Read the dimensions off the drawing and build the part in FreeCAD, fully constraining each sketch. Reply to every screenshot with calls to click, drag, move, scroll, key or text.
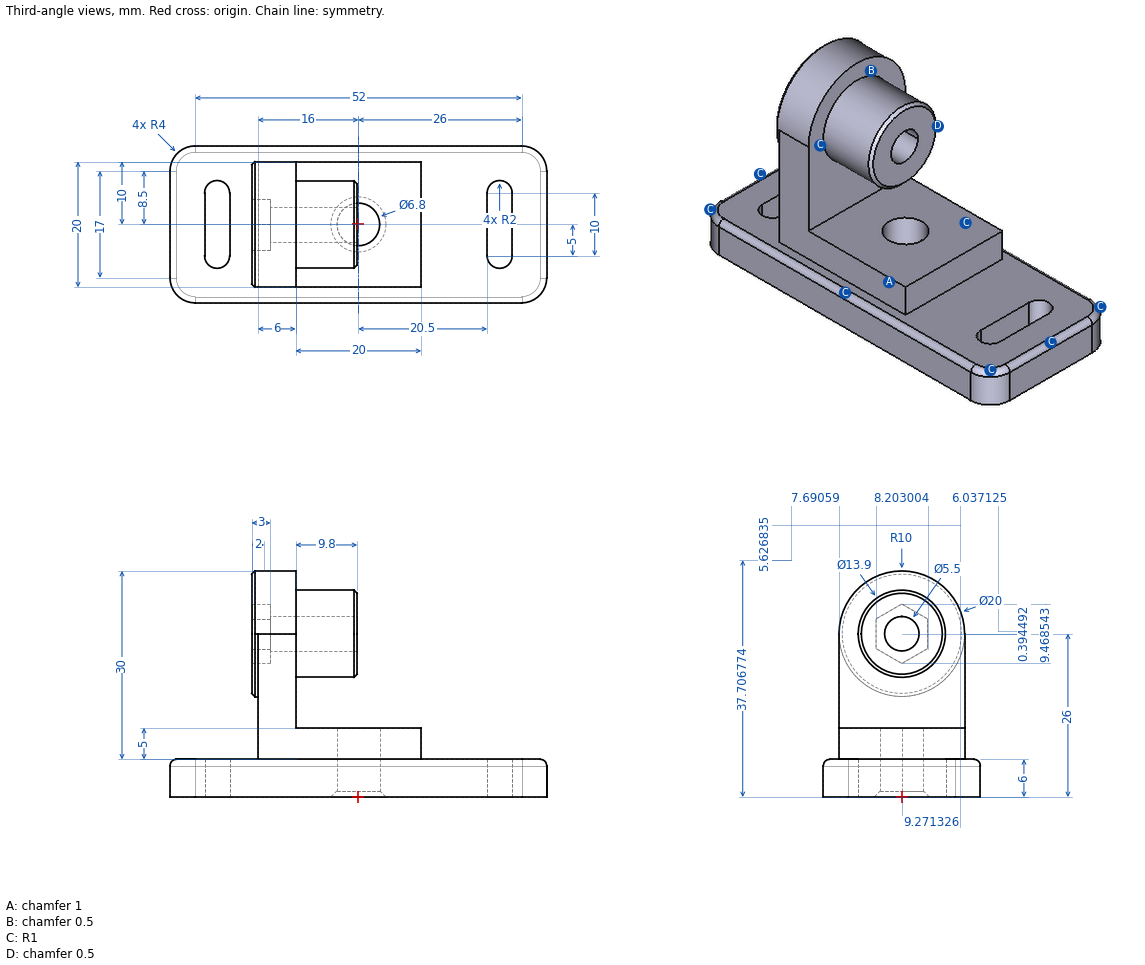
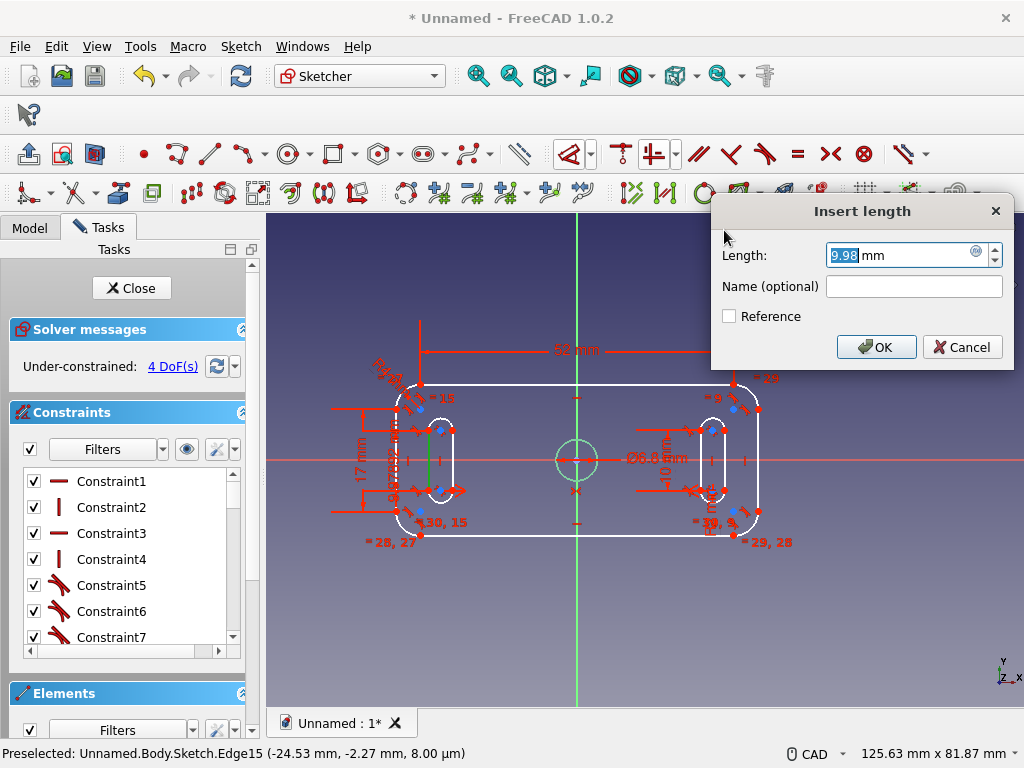
text(10)
key(Return)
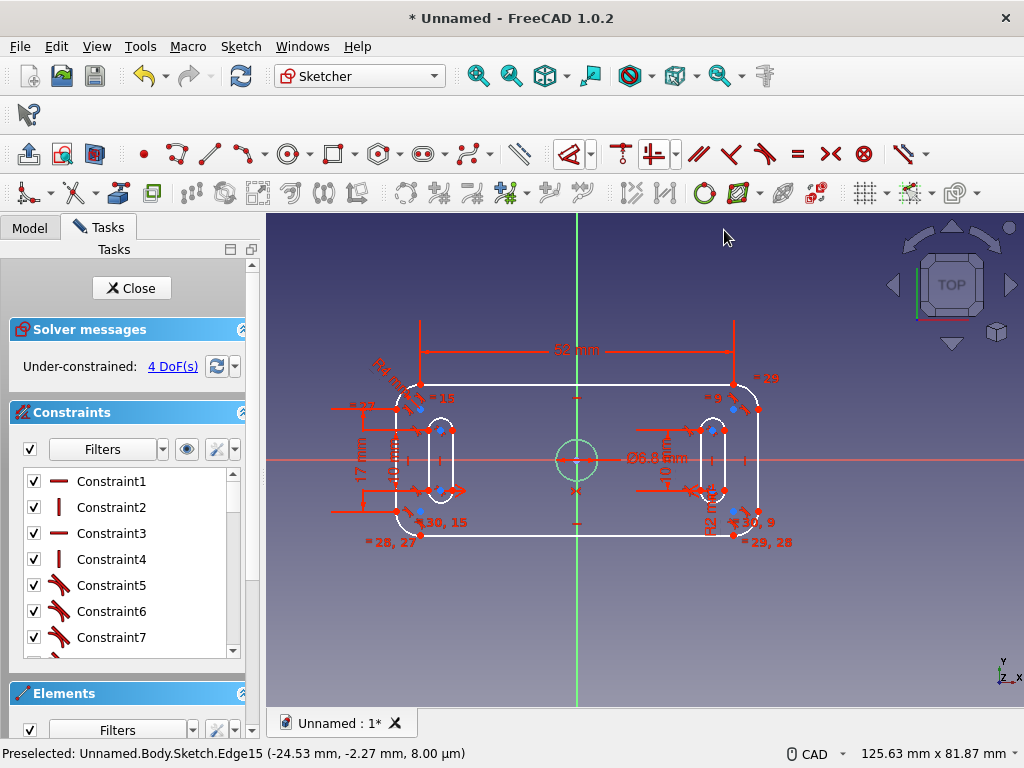
scroll(701, 491, up, 2)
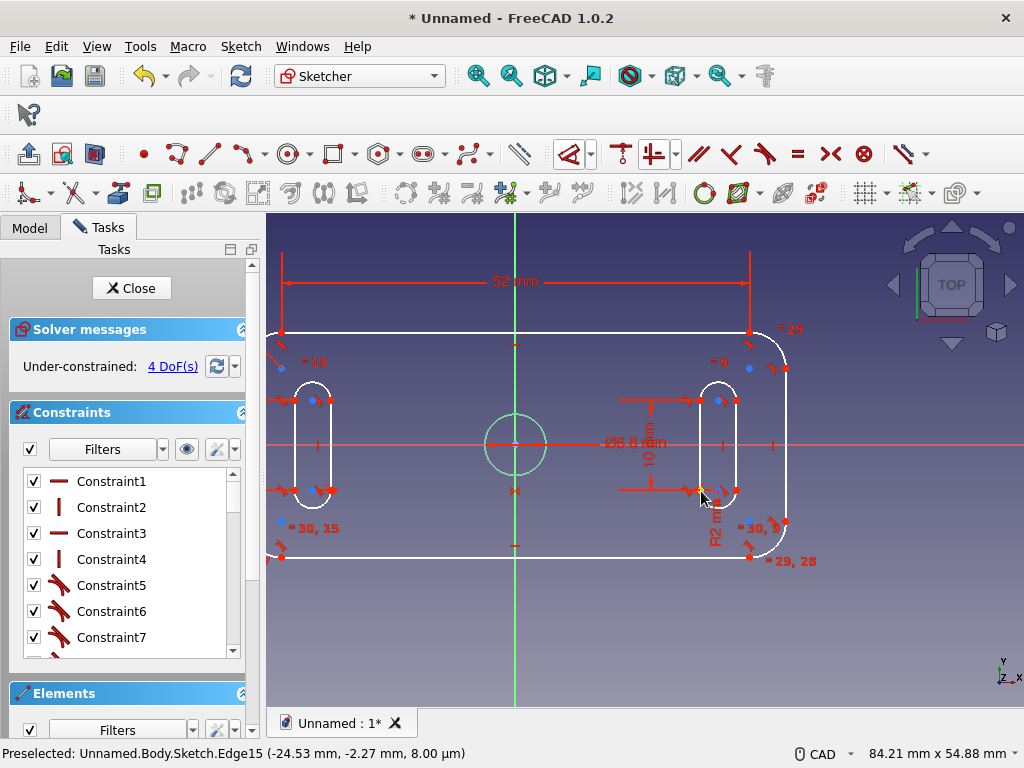
click(700, 490)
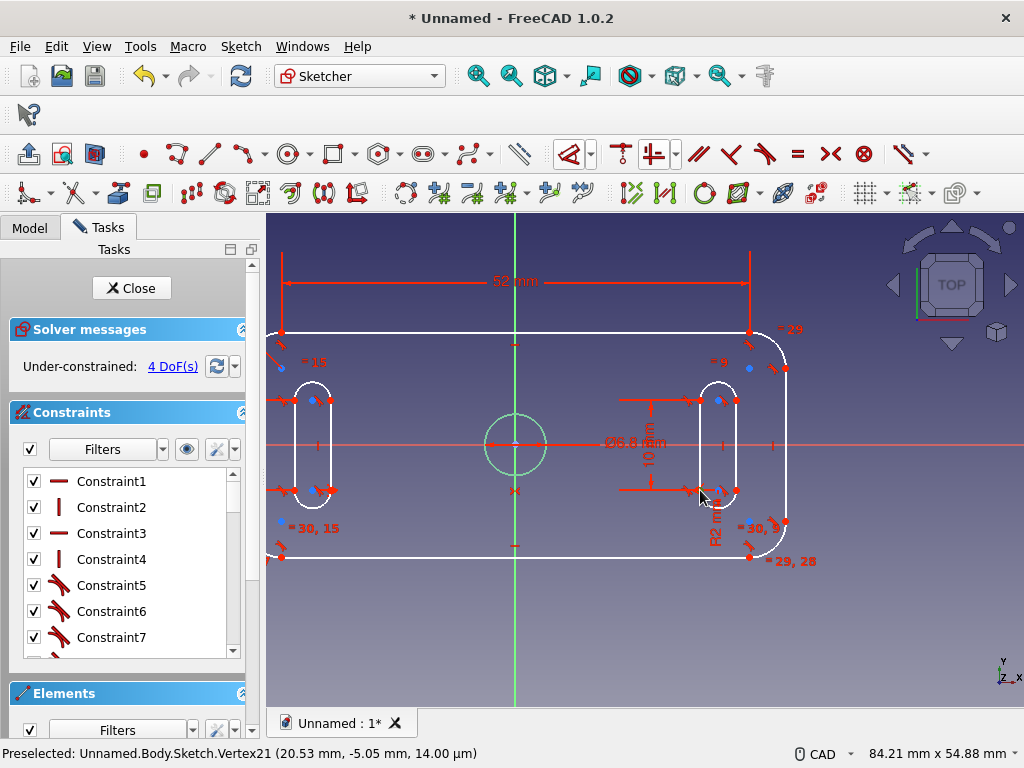
key(i)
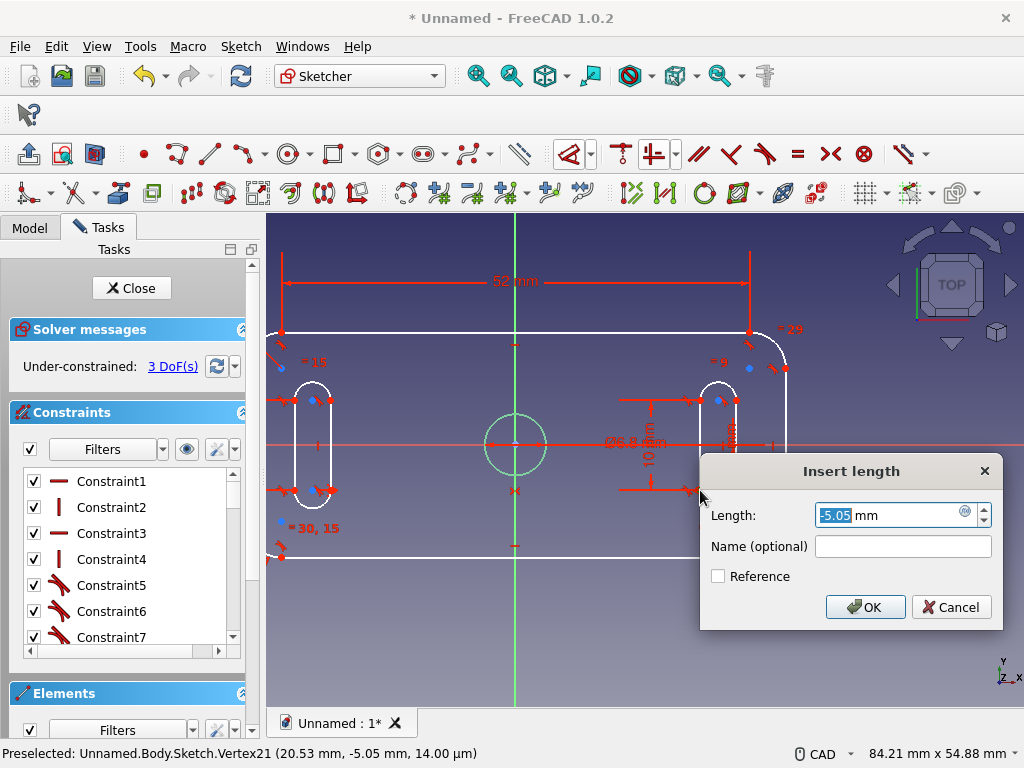
text(-5)
key(Return)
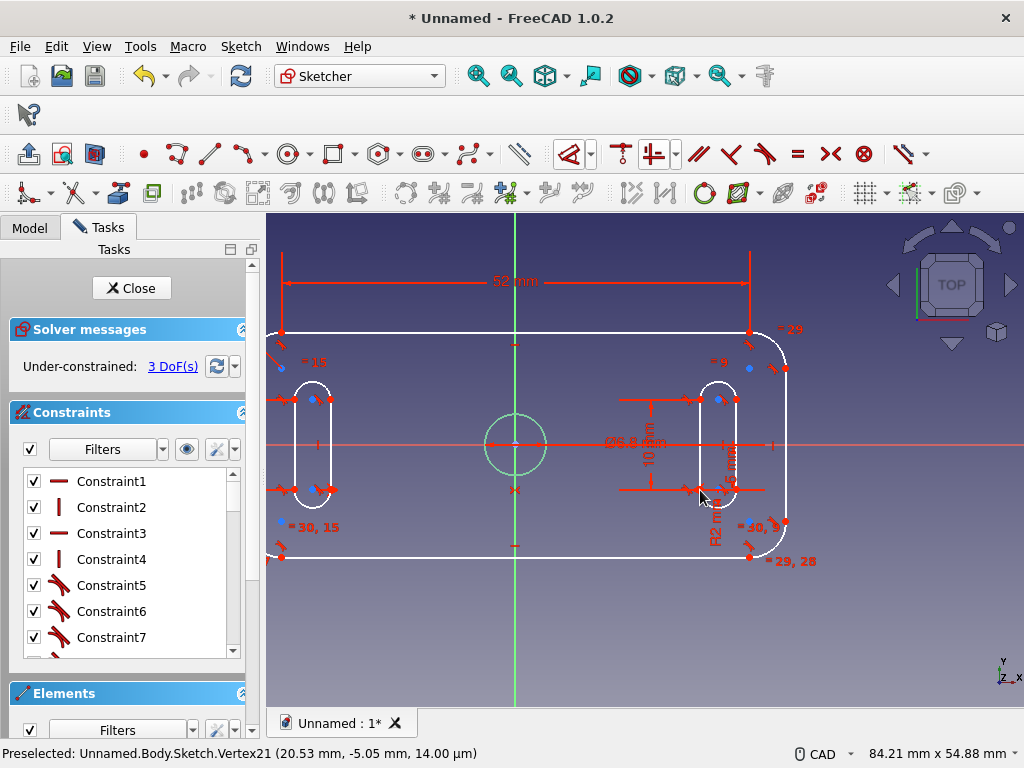
click(750, 333)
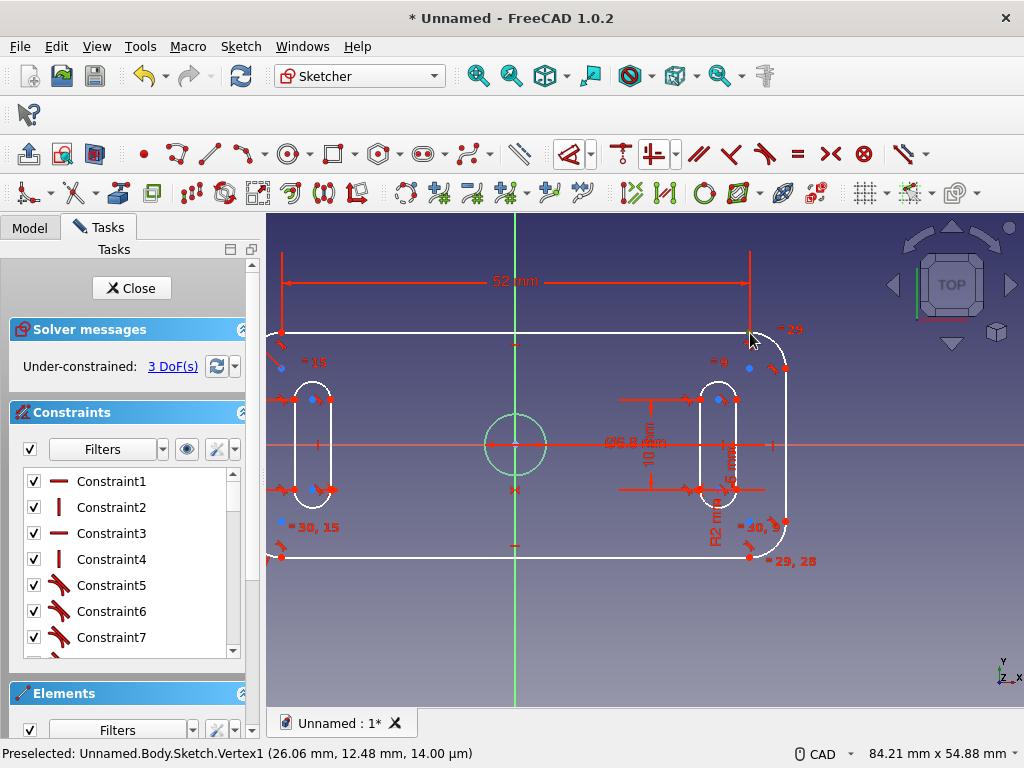
key(l)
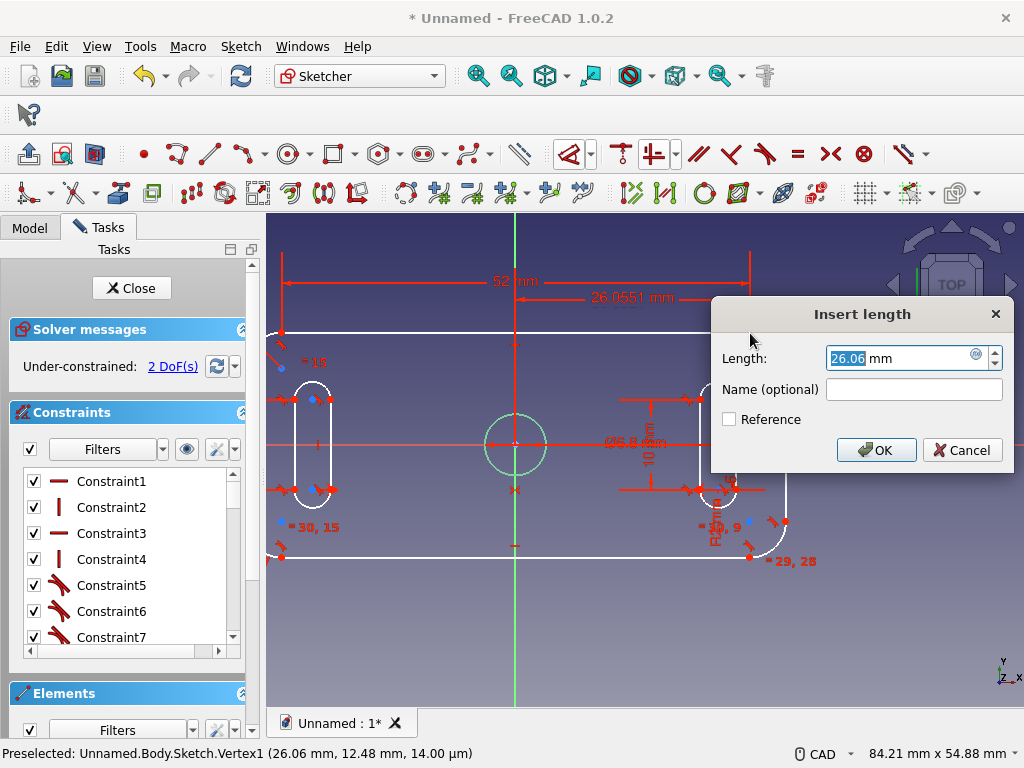
text(26)
key(Return)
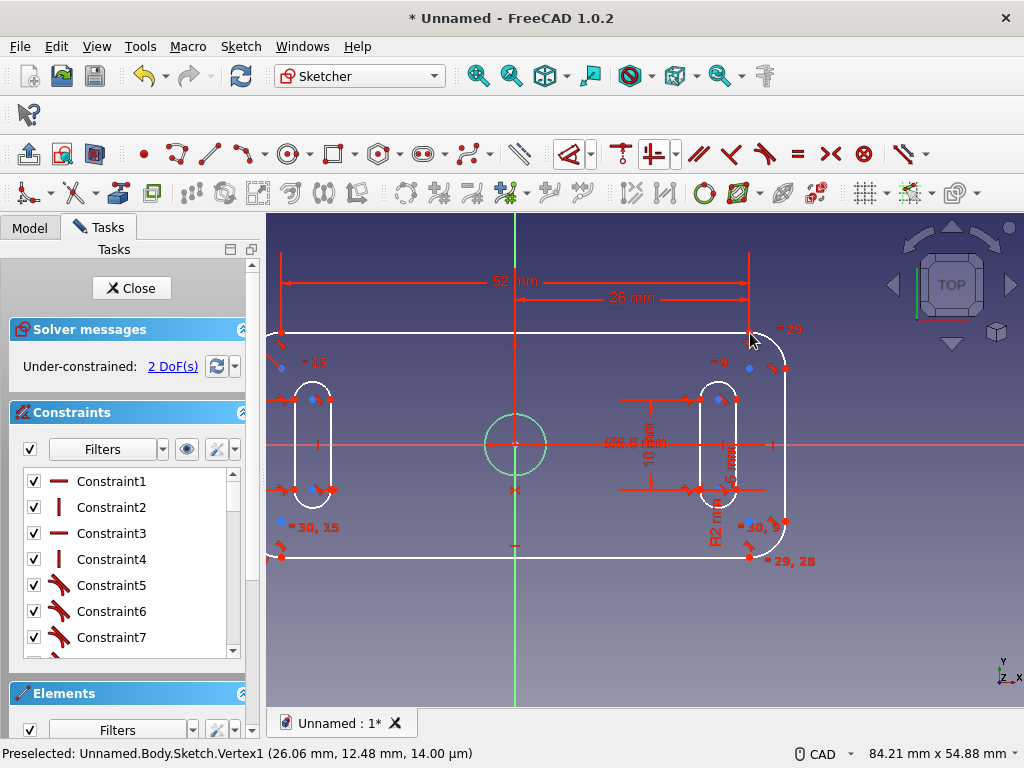
scroll(701, 491, down, 2)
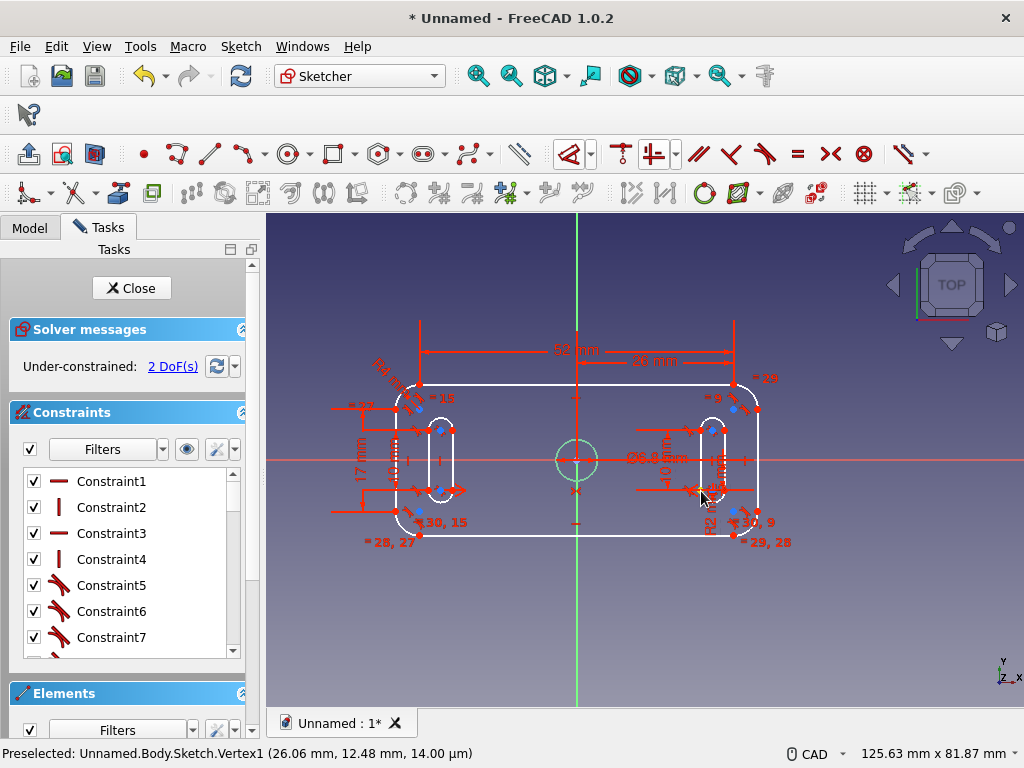
click(396, 409)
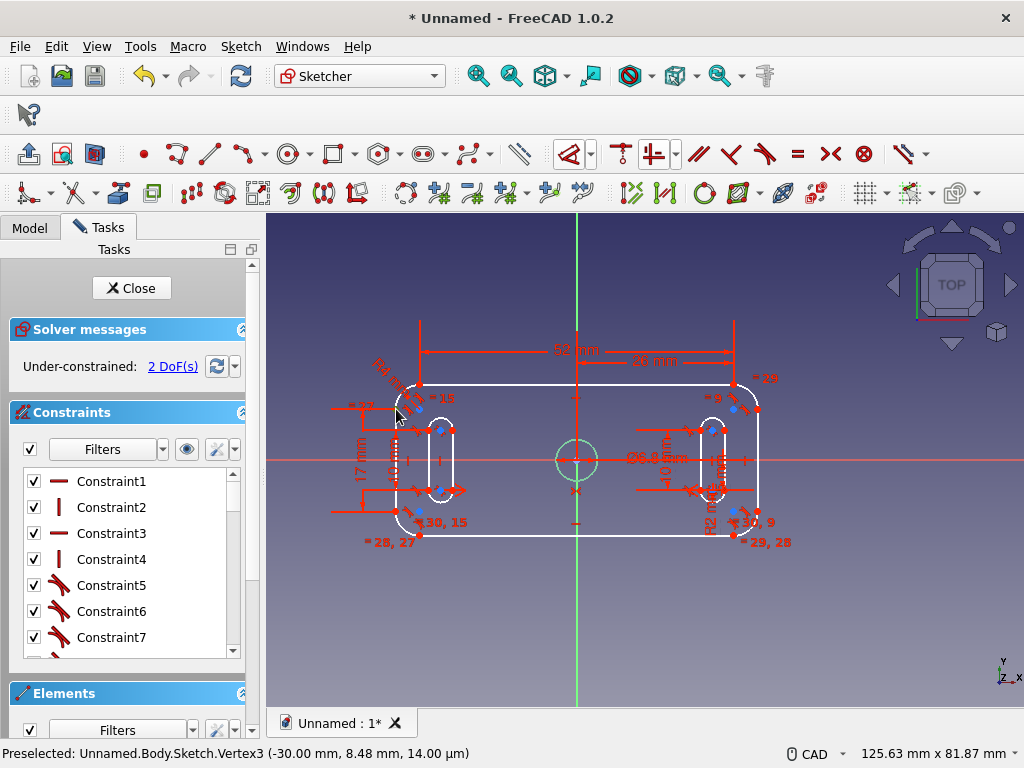
key(i)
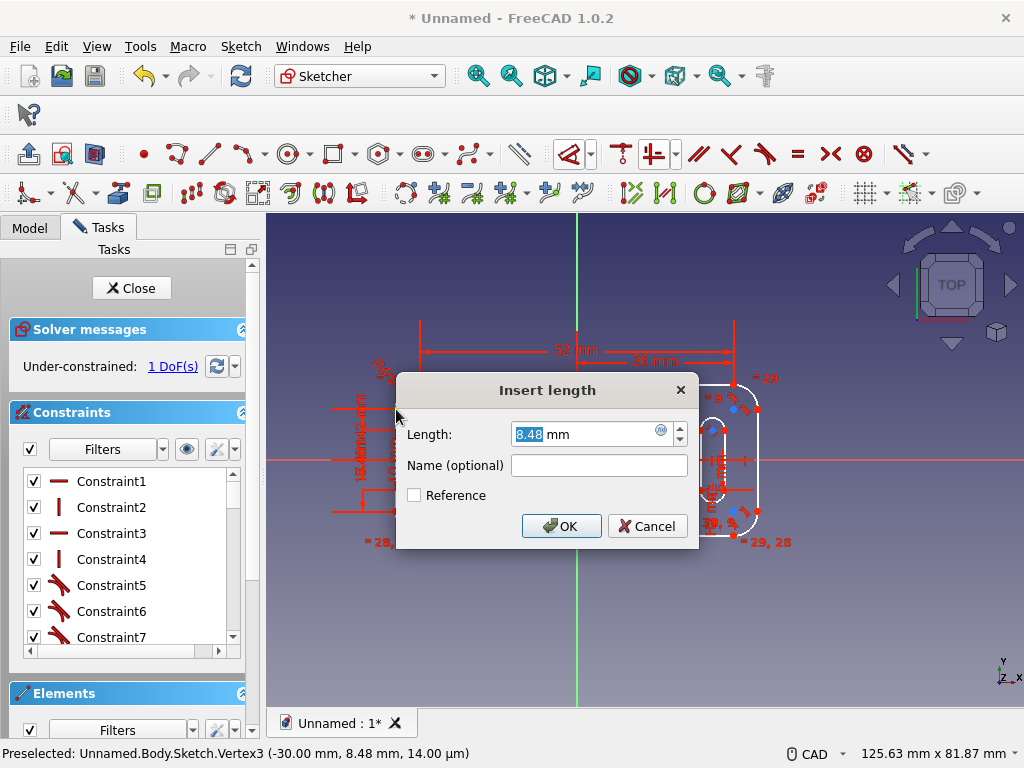
text(8.5)
key(Return)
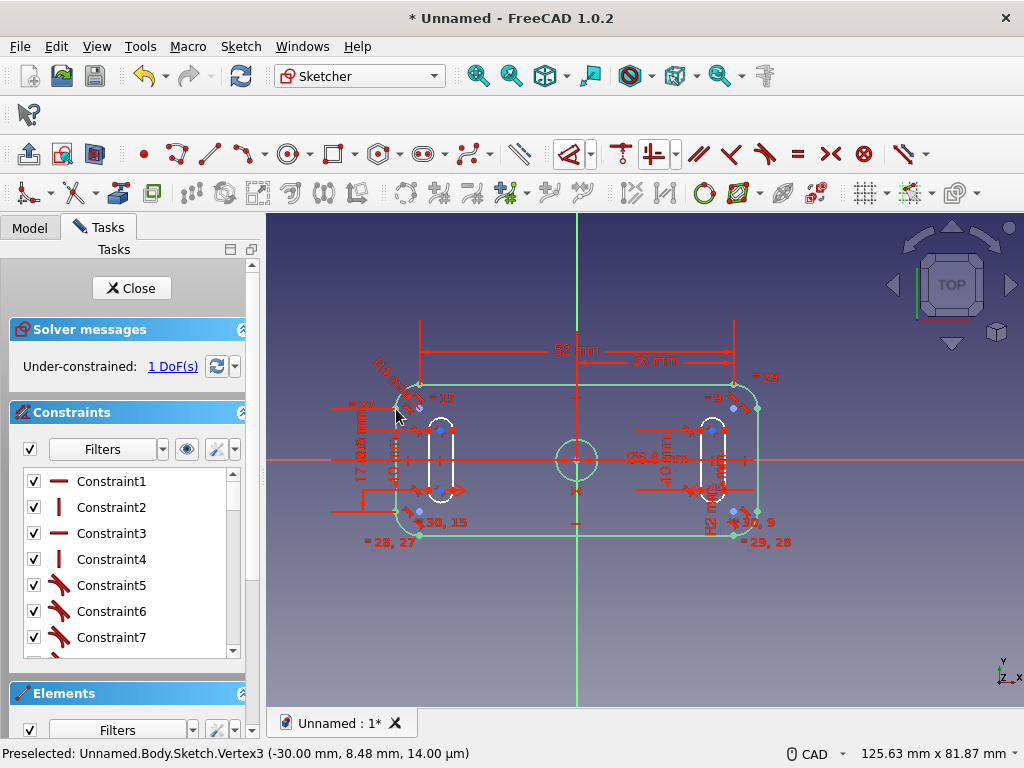
click(701, 490)